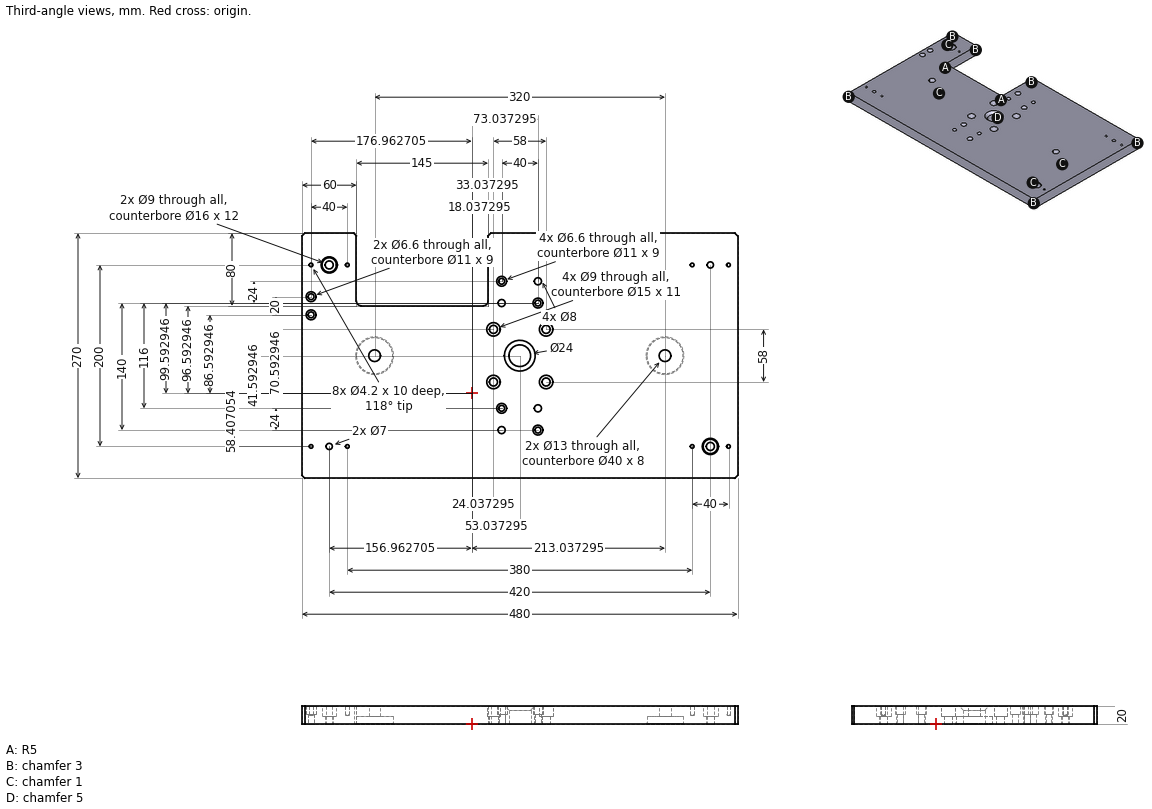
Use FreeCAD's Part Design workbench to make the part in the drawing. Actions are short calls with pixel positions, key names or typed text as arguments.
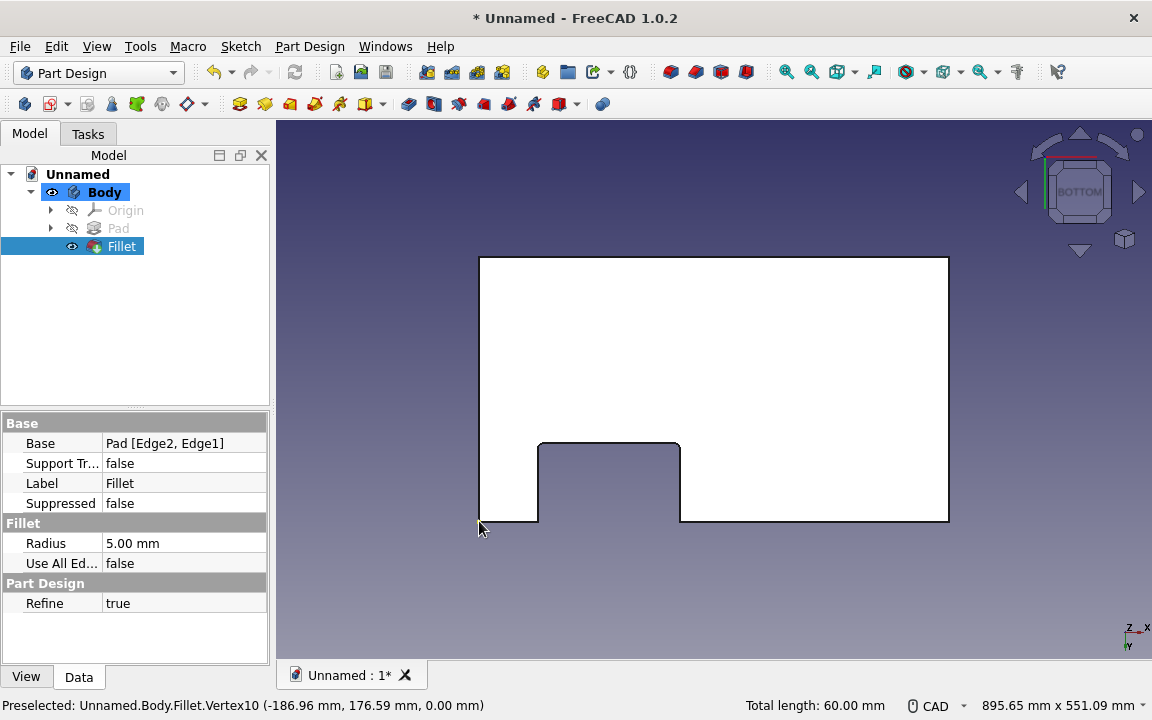
key(4)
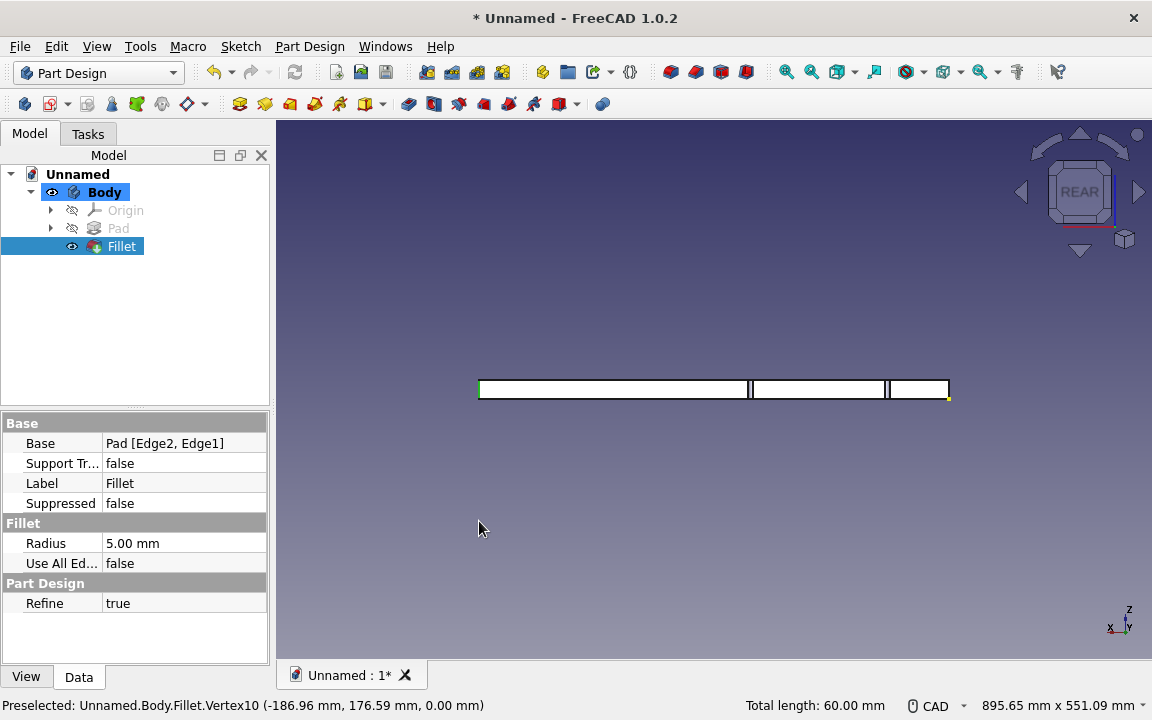
click(949, 388, ctrl)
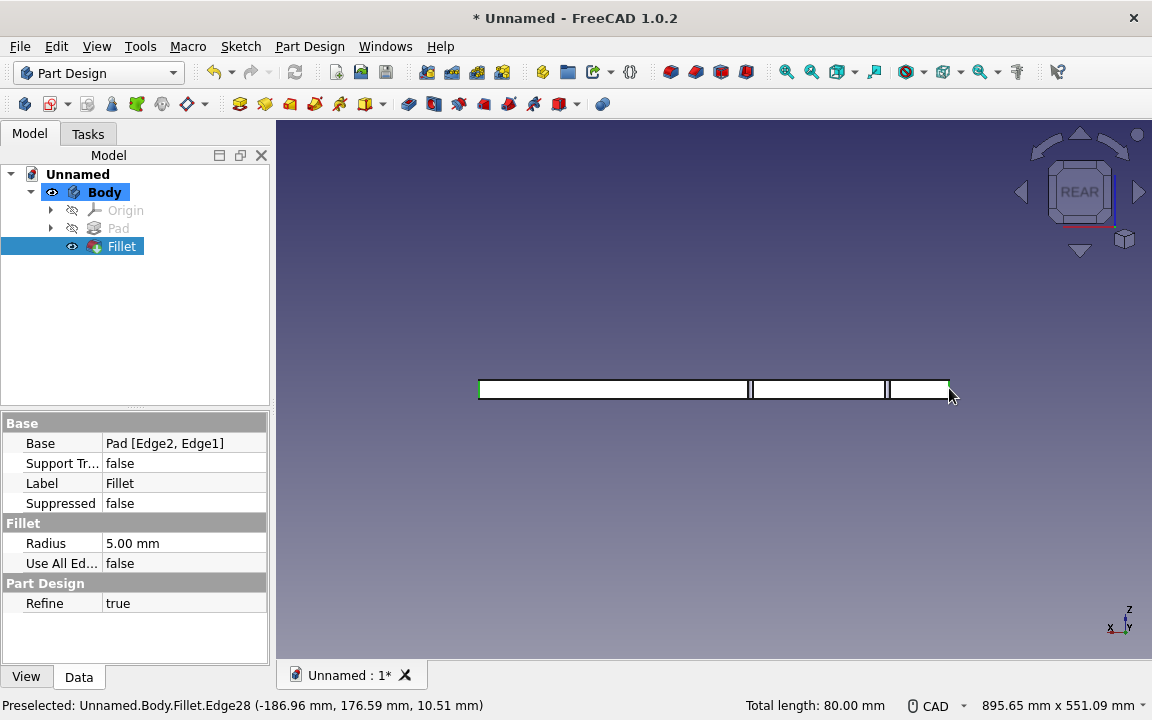
click(890, 388, ctrl)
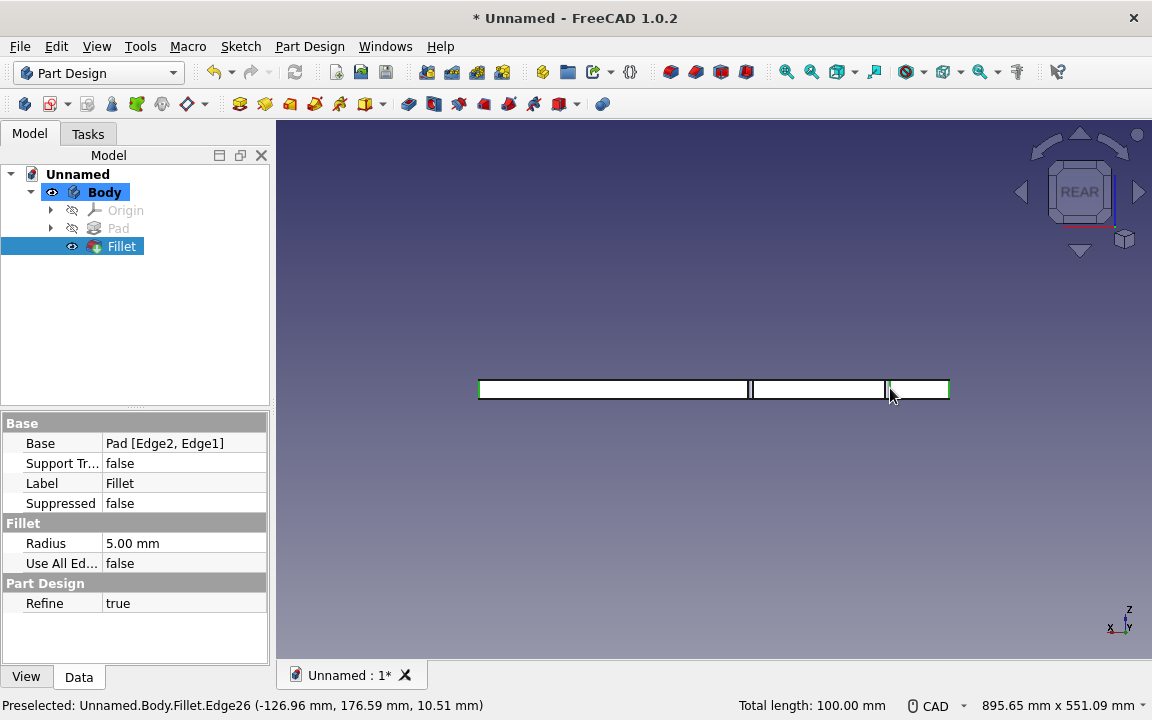
click(748, 388, ctrl)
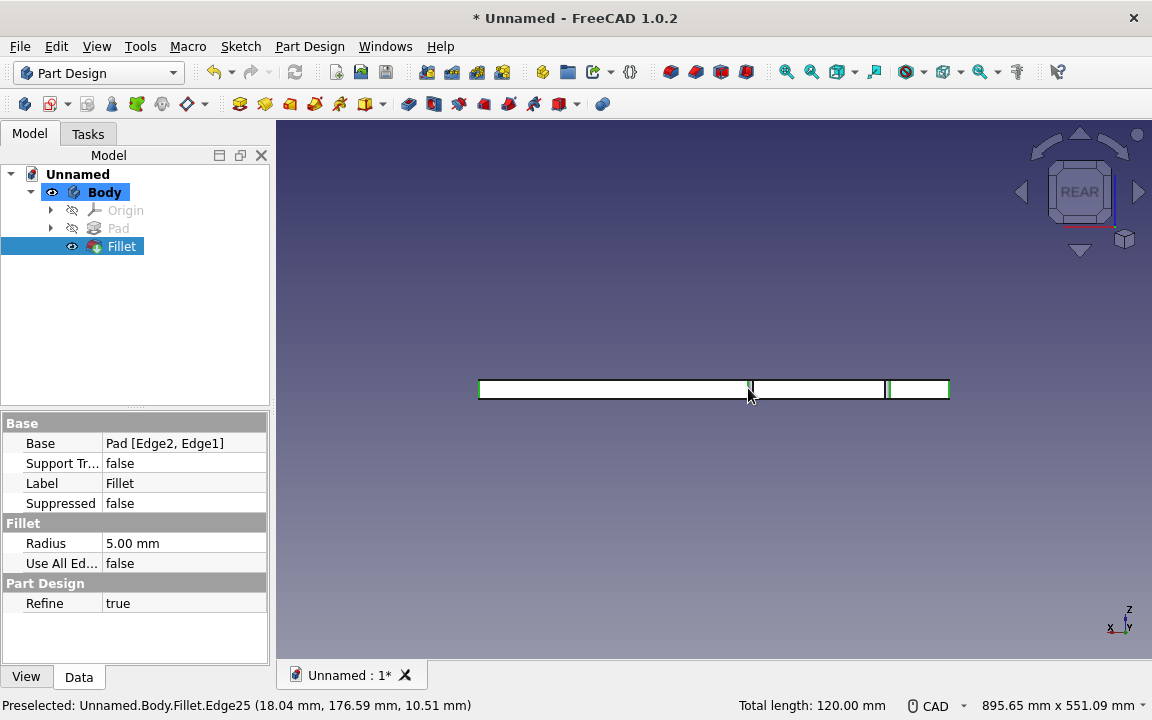
click(696, 72)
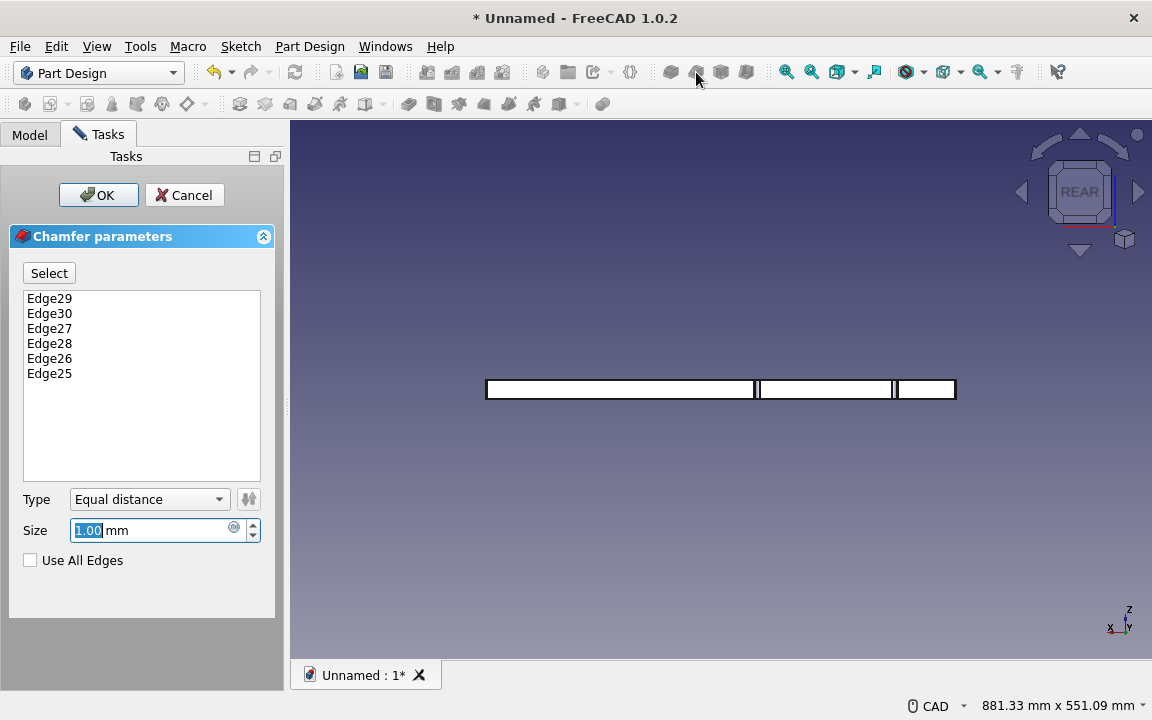
text(3)
key(Tab)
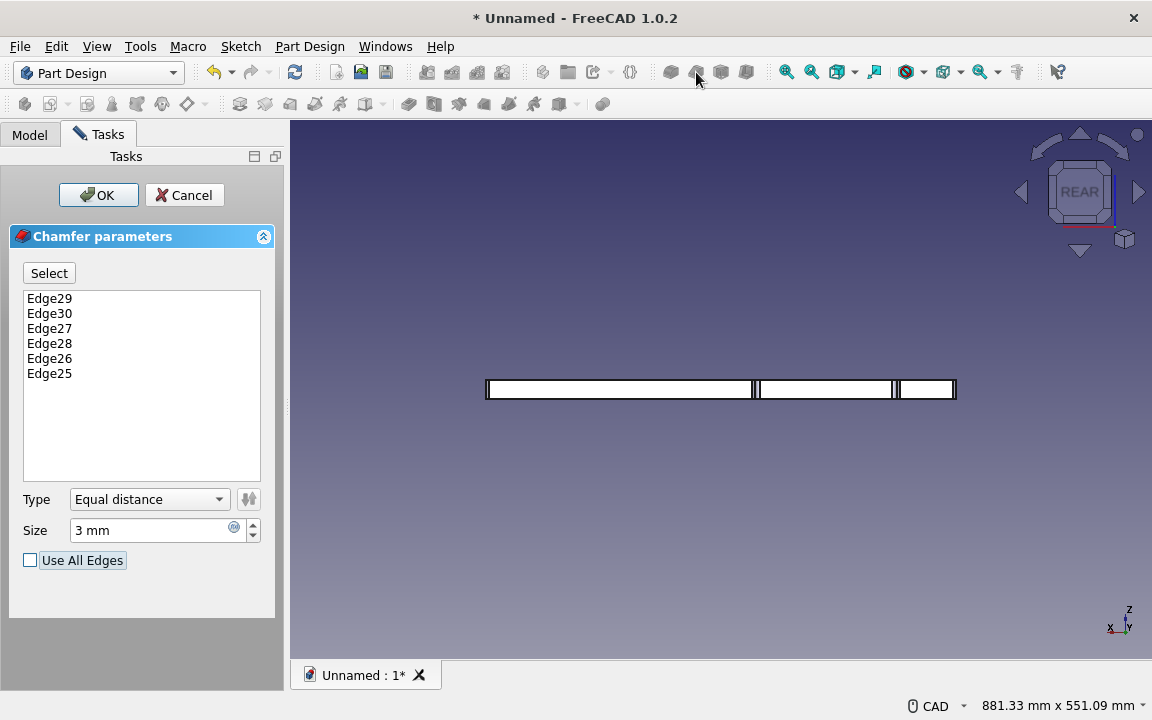
click(99, 195)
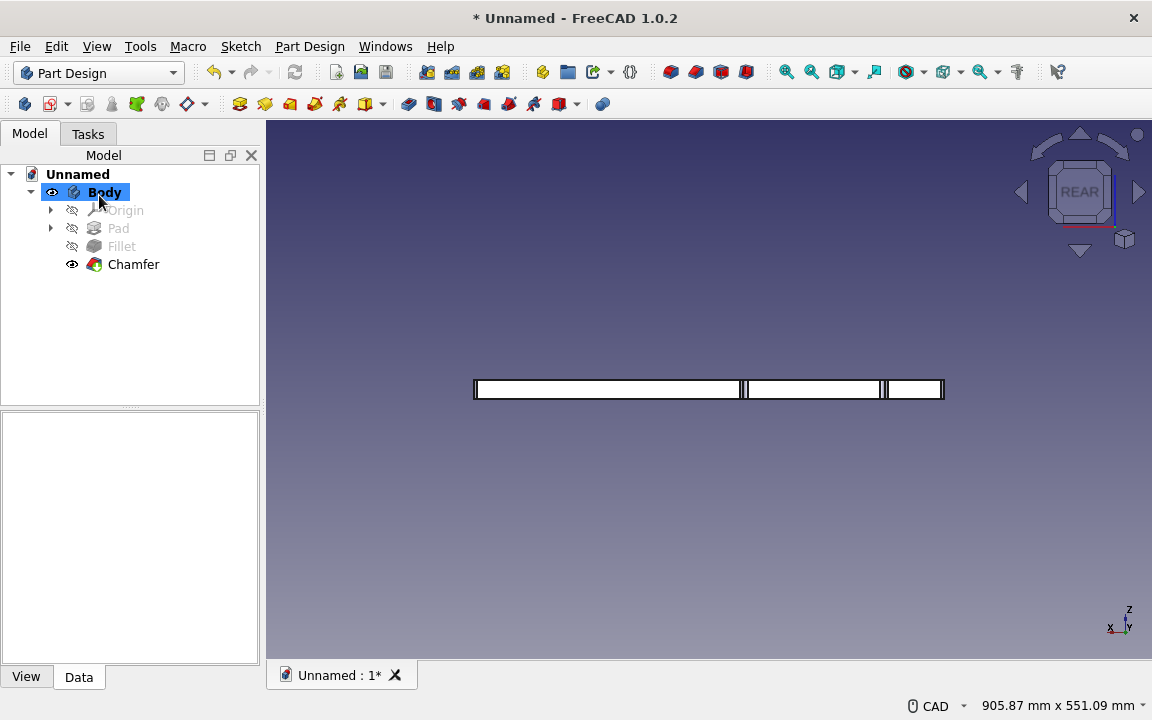
key(0)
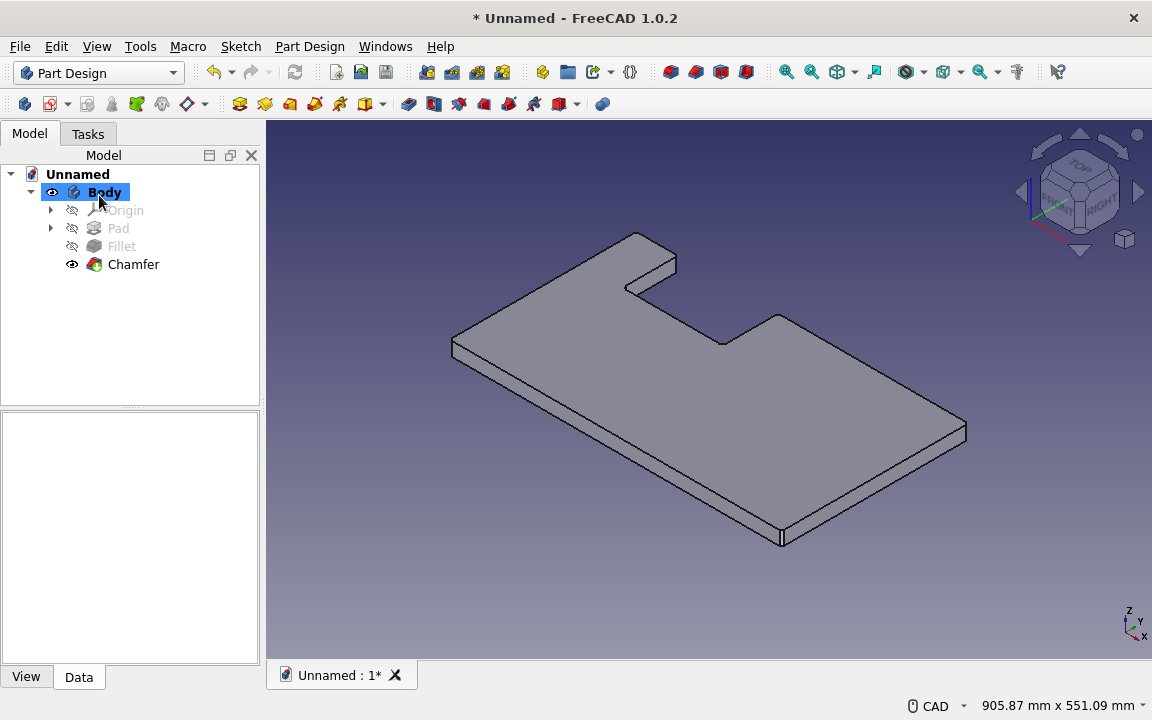
click(756, 408)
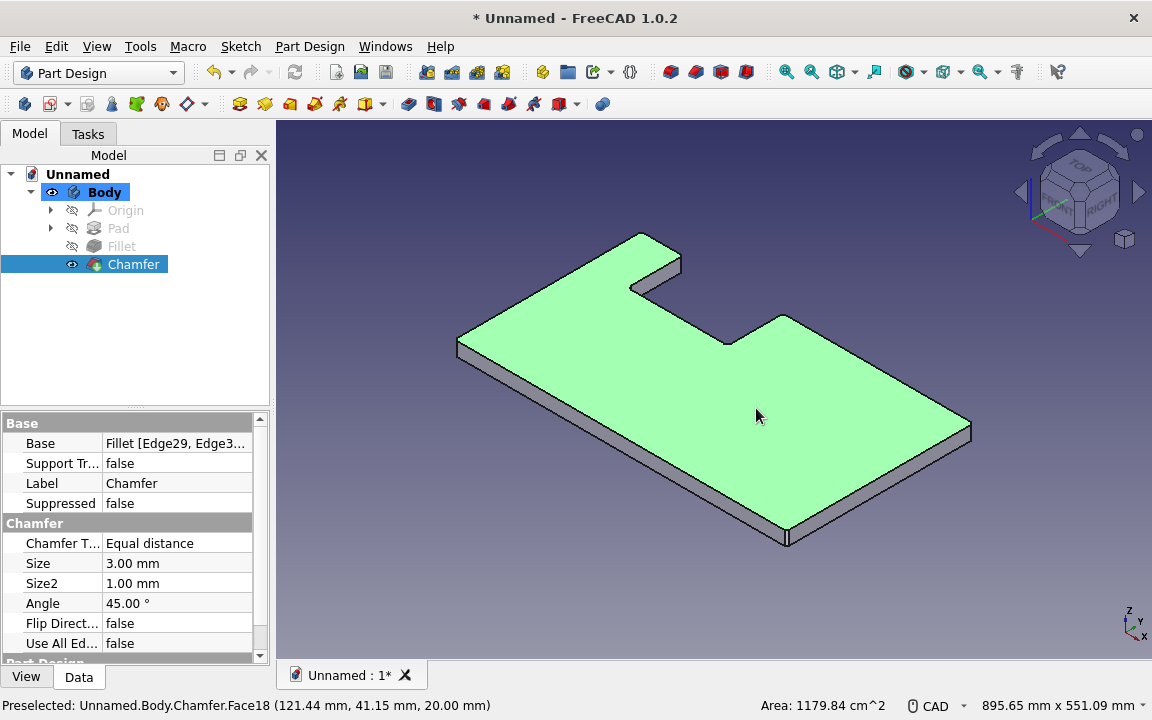
click(50, 104)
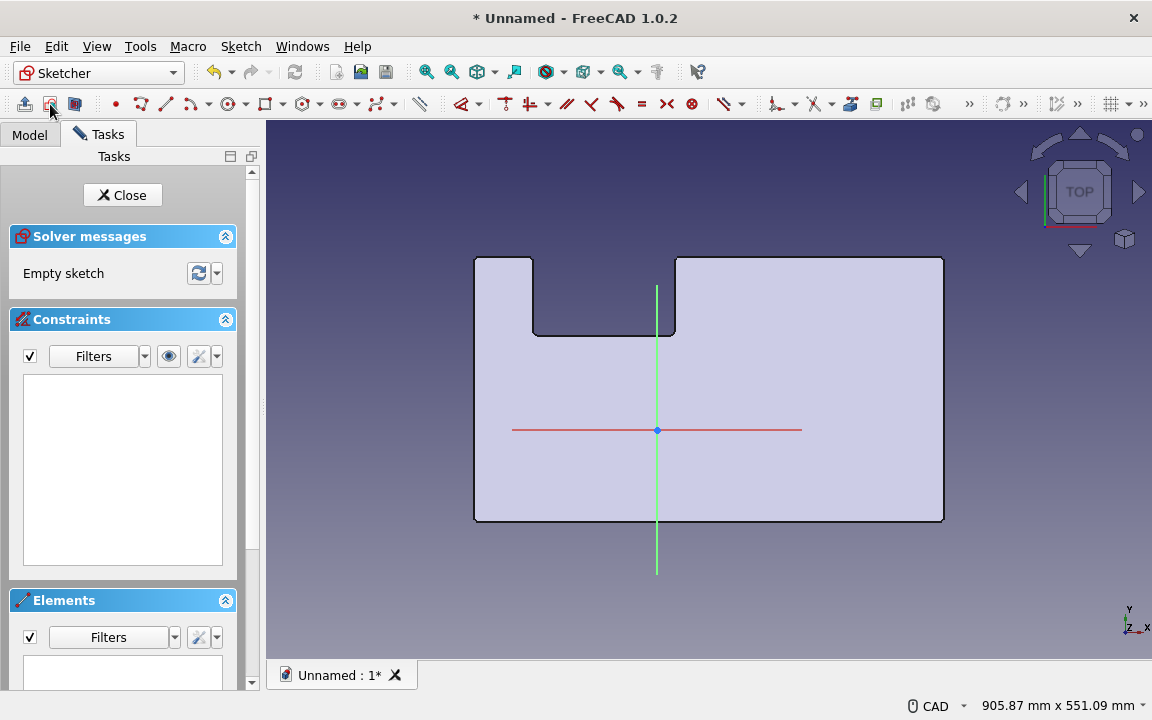
scroll(471, 331, up, 13)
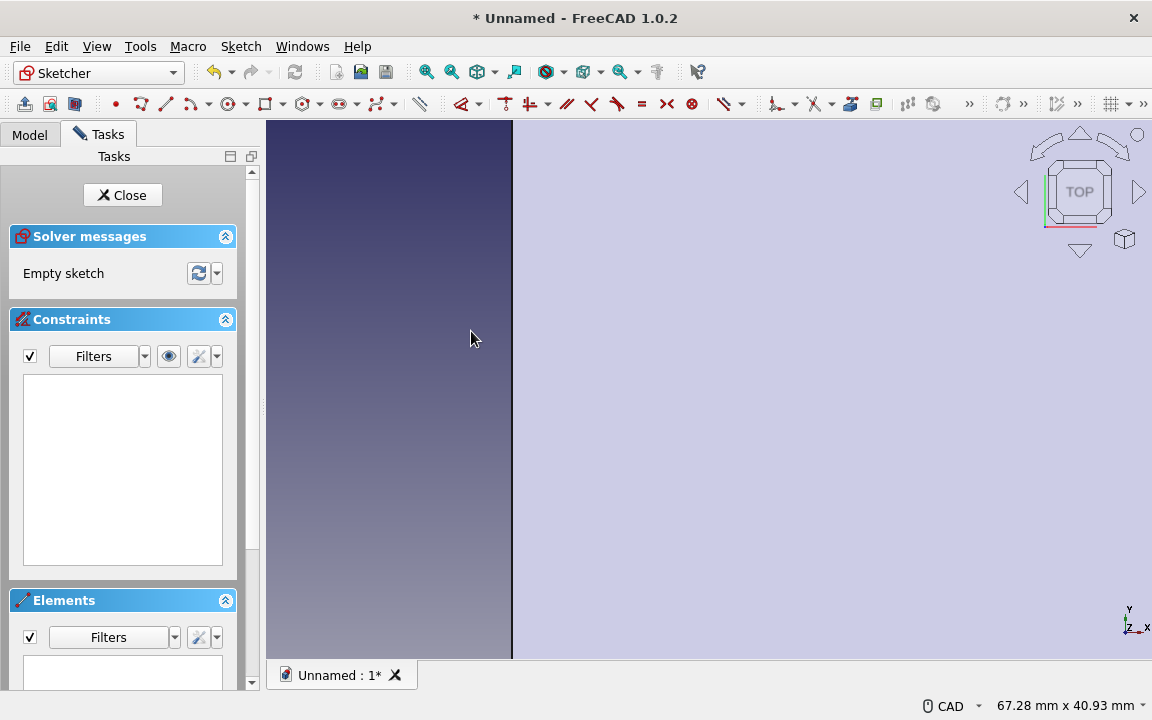
key(g)
key(c)